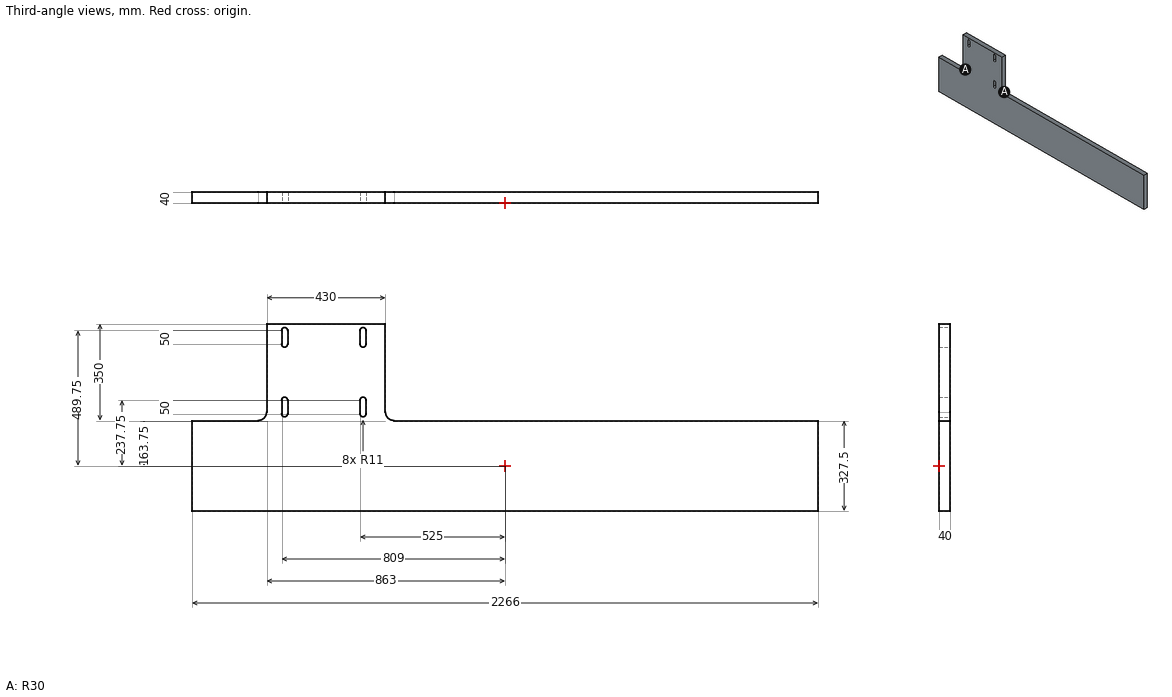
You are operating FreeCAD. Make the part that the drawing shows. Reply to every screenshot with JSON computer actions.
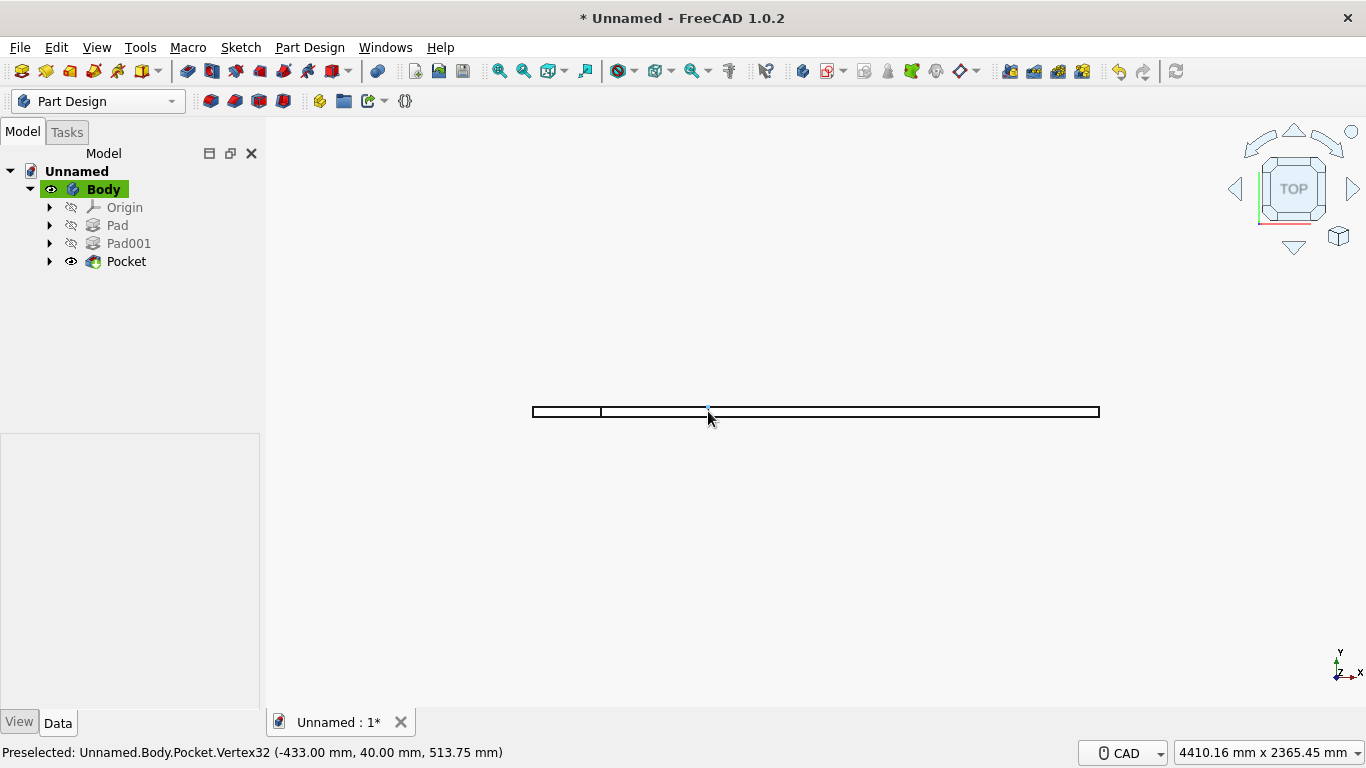
{"action": "key", "text": "1"}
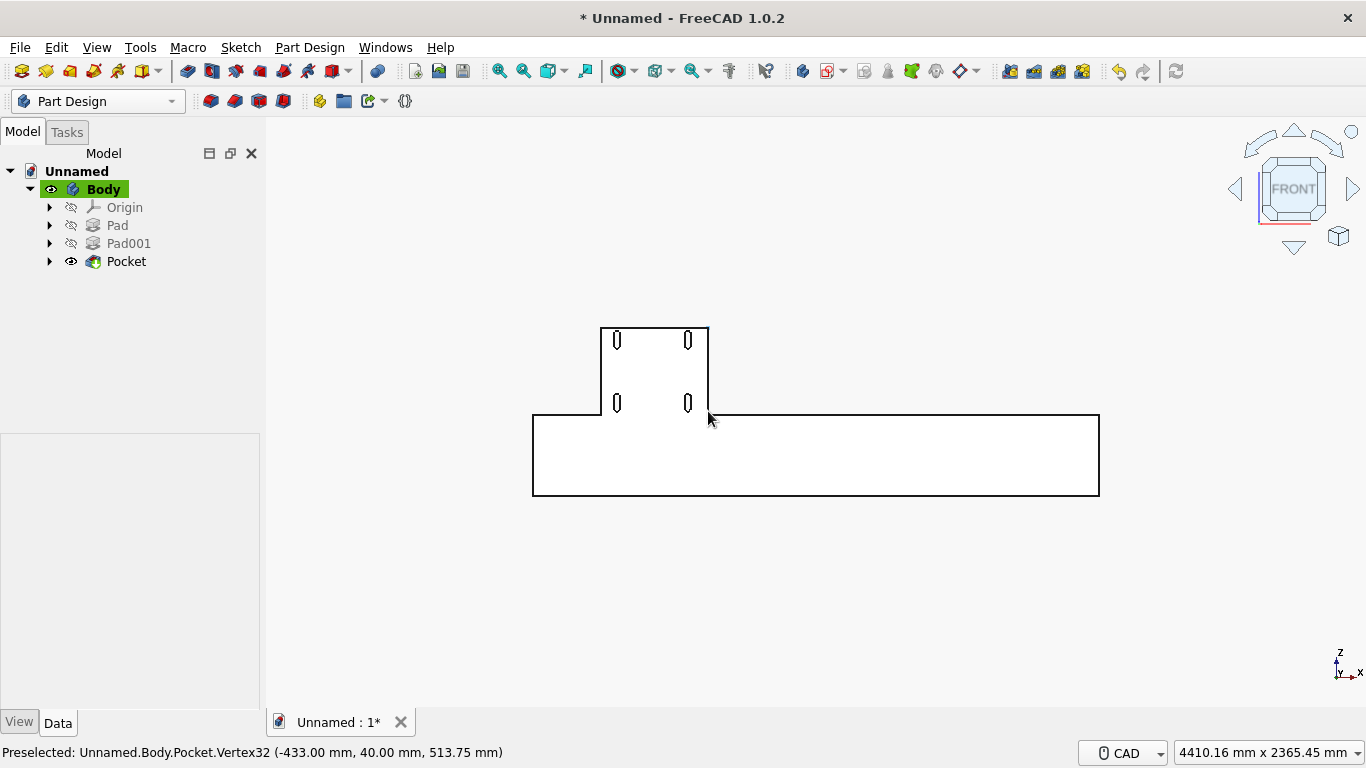
{"action": "scroll", "coordinate": [708, 414], "scroll_direction": "up", "scroll_amount": 7}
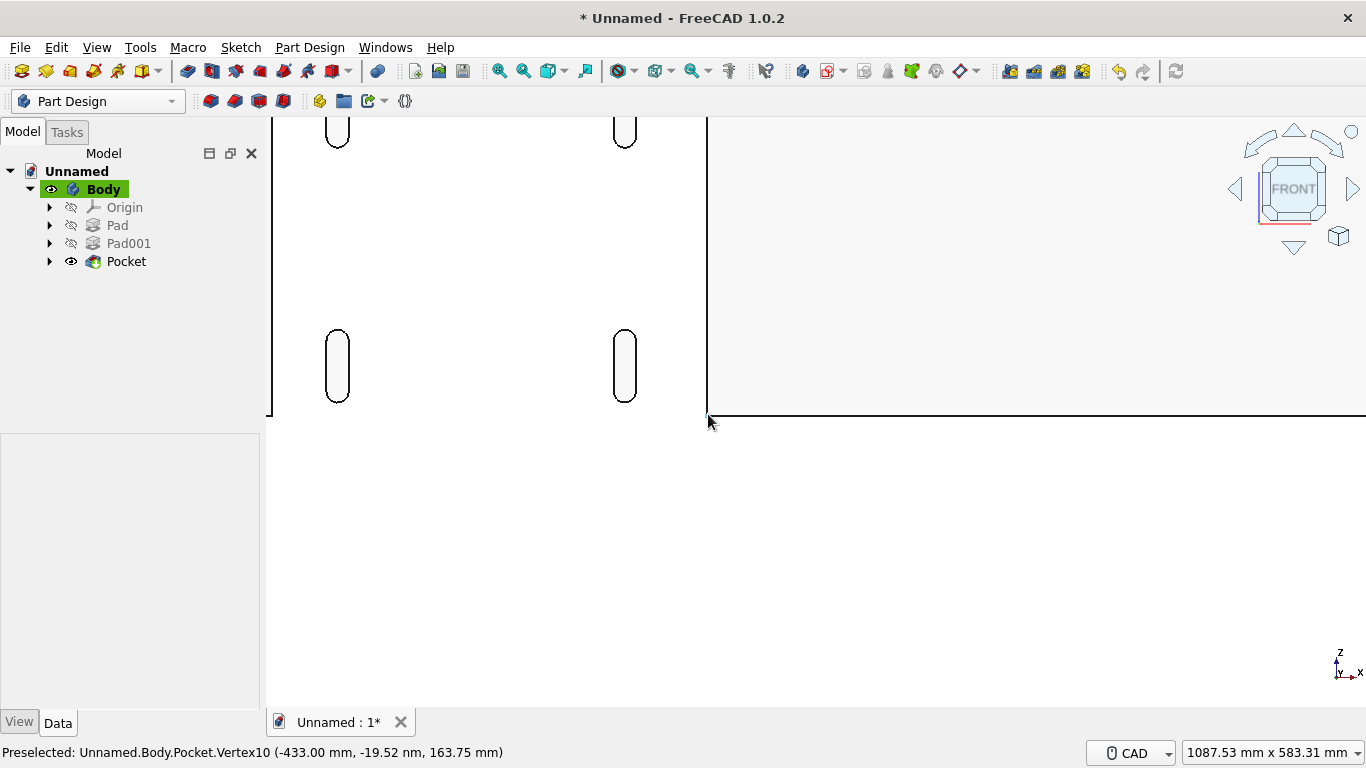
{"action": "left_click", "coordinate": [500, 72]}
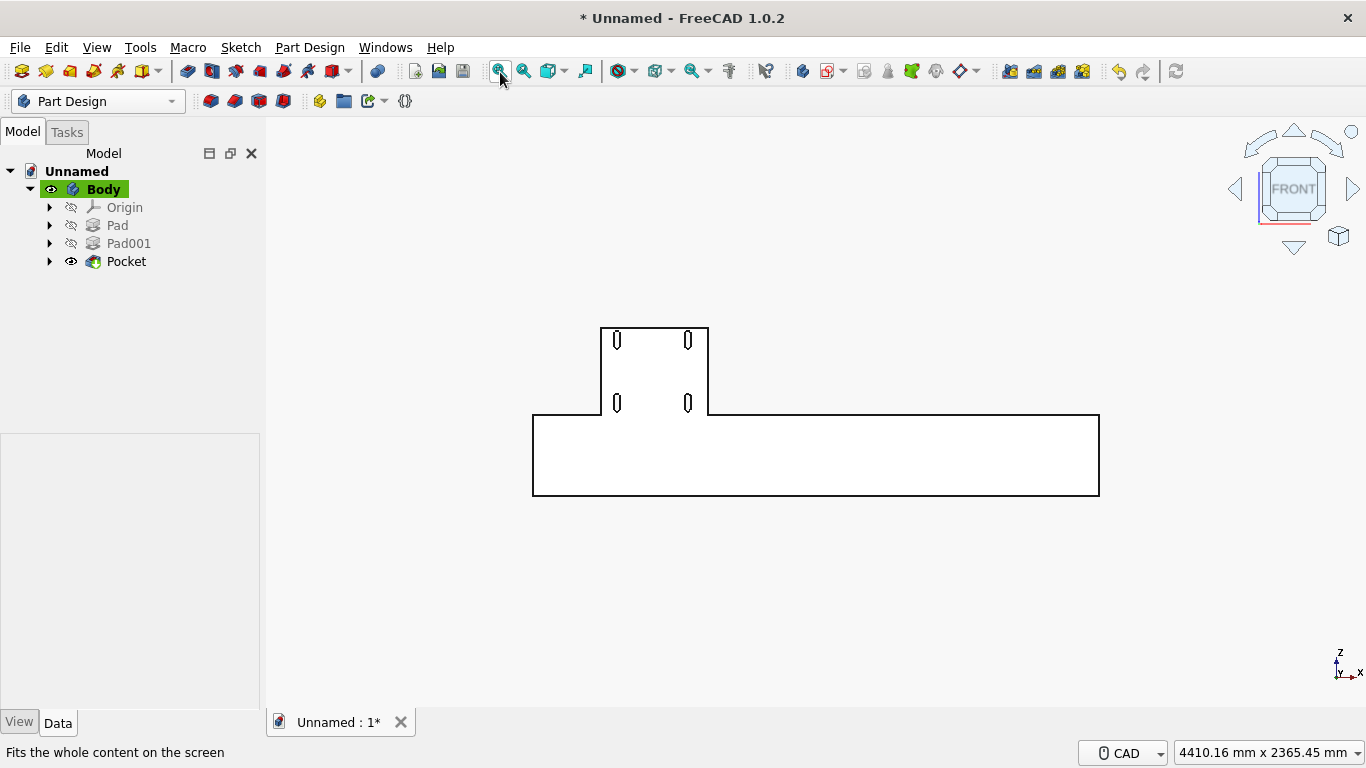
{"action": "key", "text": "3"}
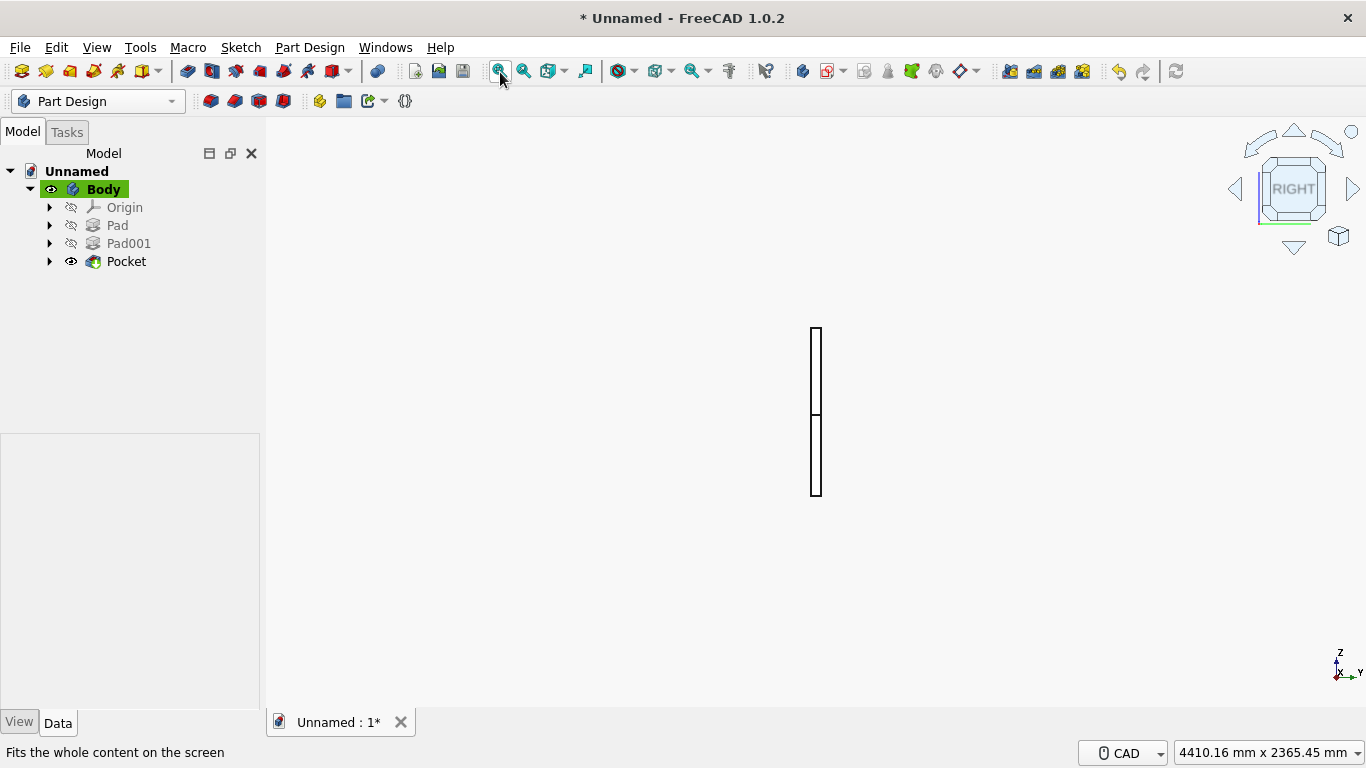
{"action": "key", "text": "v f"}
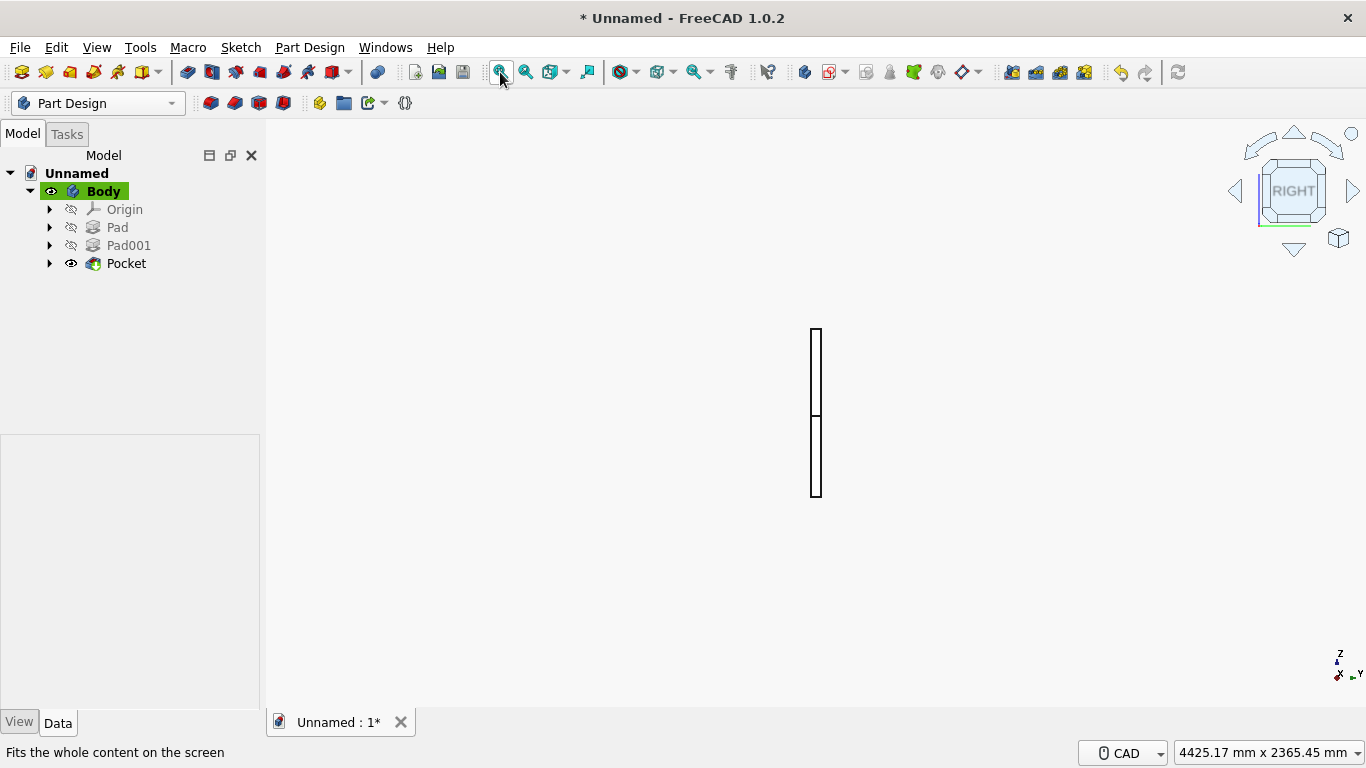
{"action": "scroll", "coordinate": [816, 415], "scroll_direction": "up", "scroll_amount": 7}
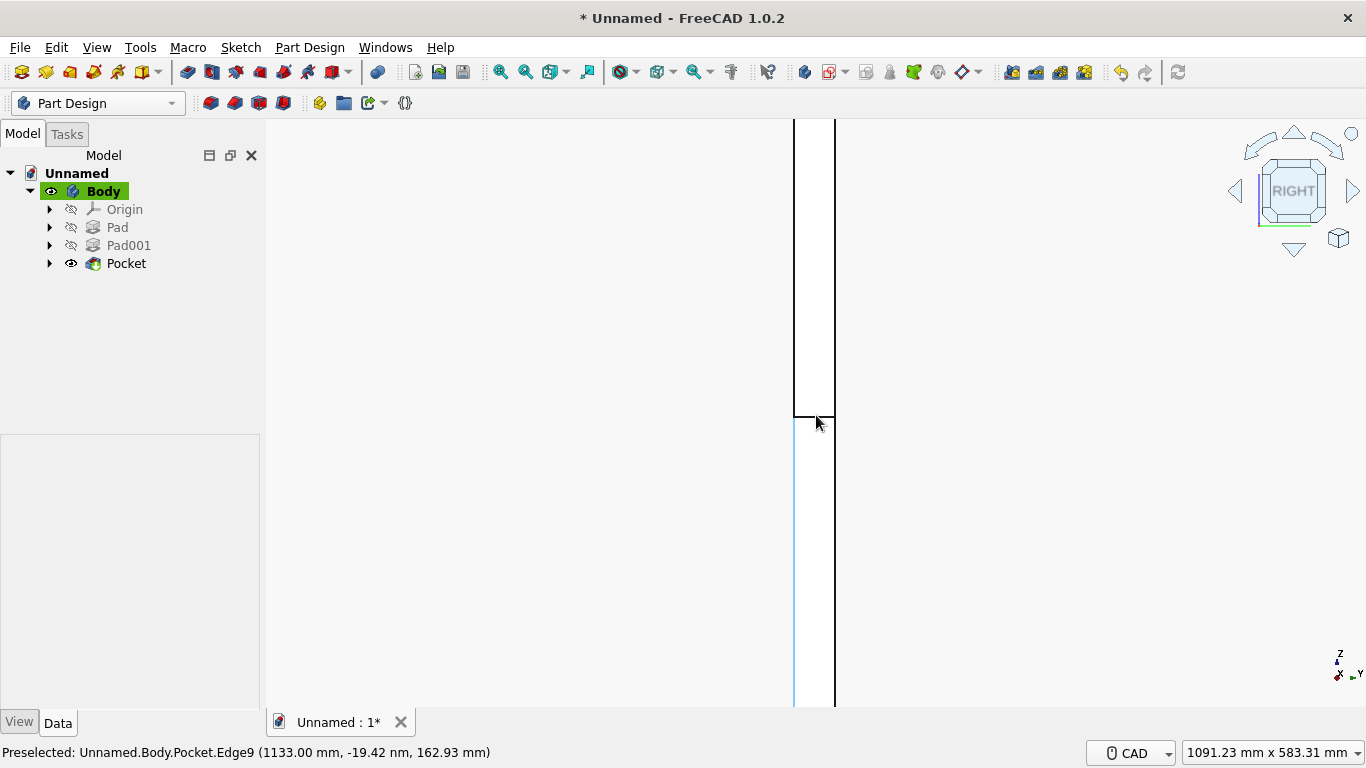
{"action": "left_click", "coordinate": [502, 72]}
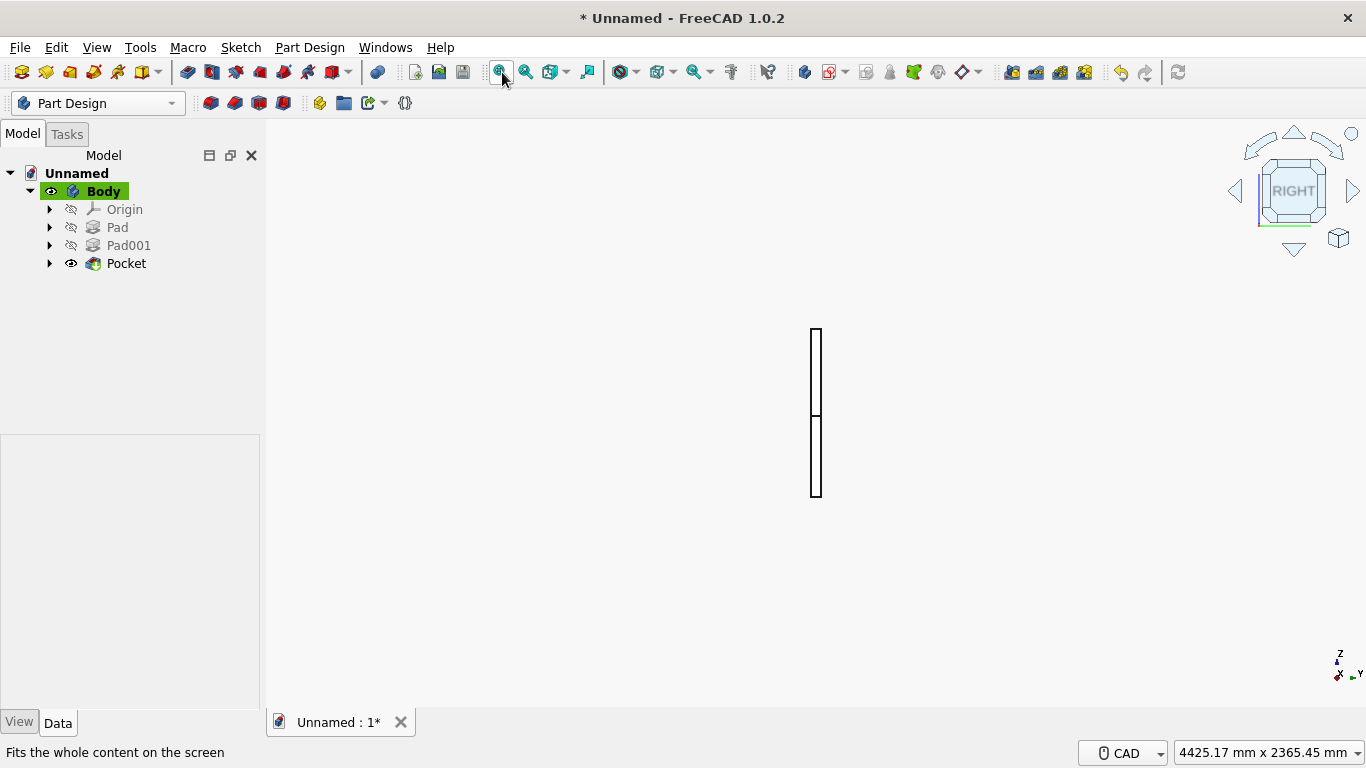
{"action": "key", "text": "5"}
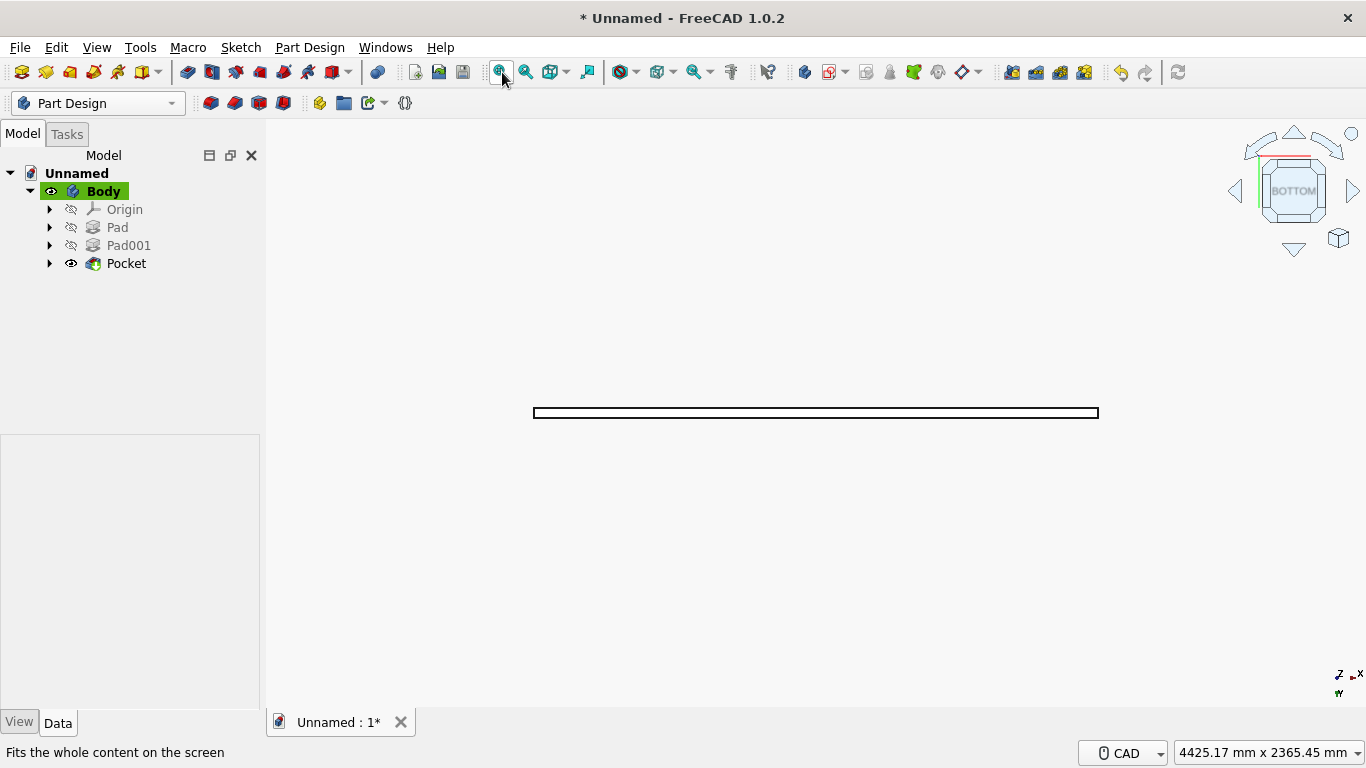
{"action": "scroll", "coordinate": [708, 412], "scroll_direction": "up", "scroll_amount": 7}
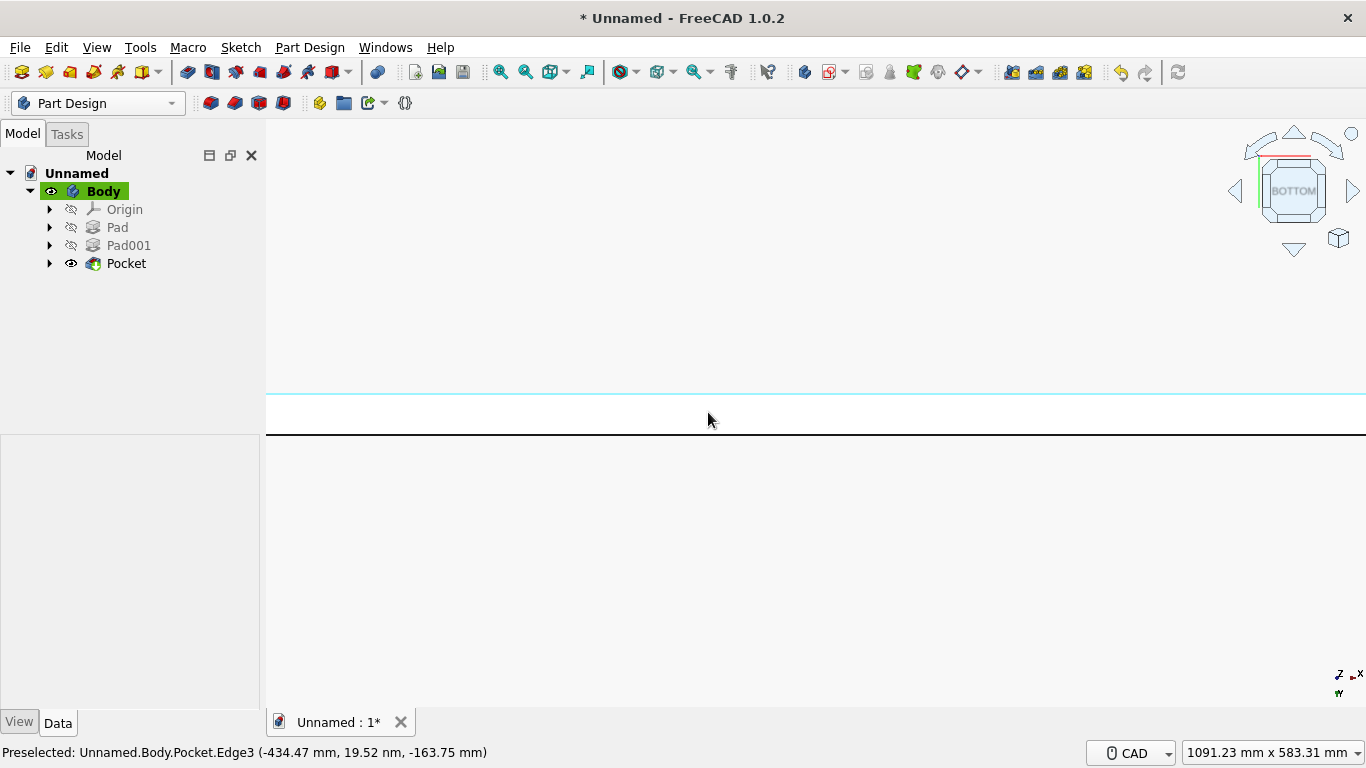
{"action": "key", "text": "v f"}